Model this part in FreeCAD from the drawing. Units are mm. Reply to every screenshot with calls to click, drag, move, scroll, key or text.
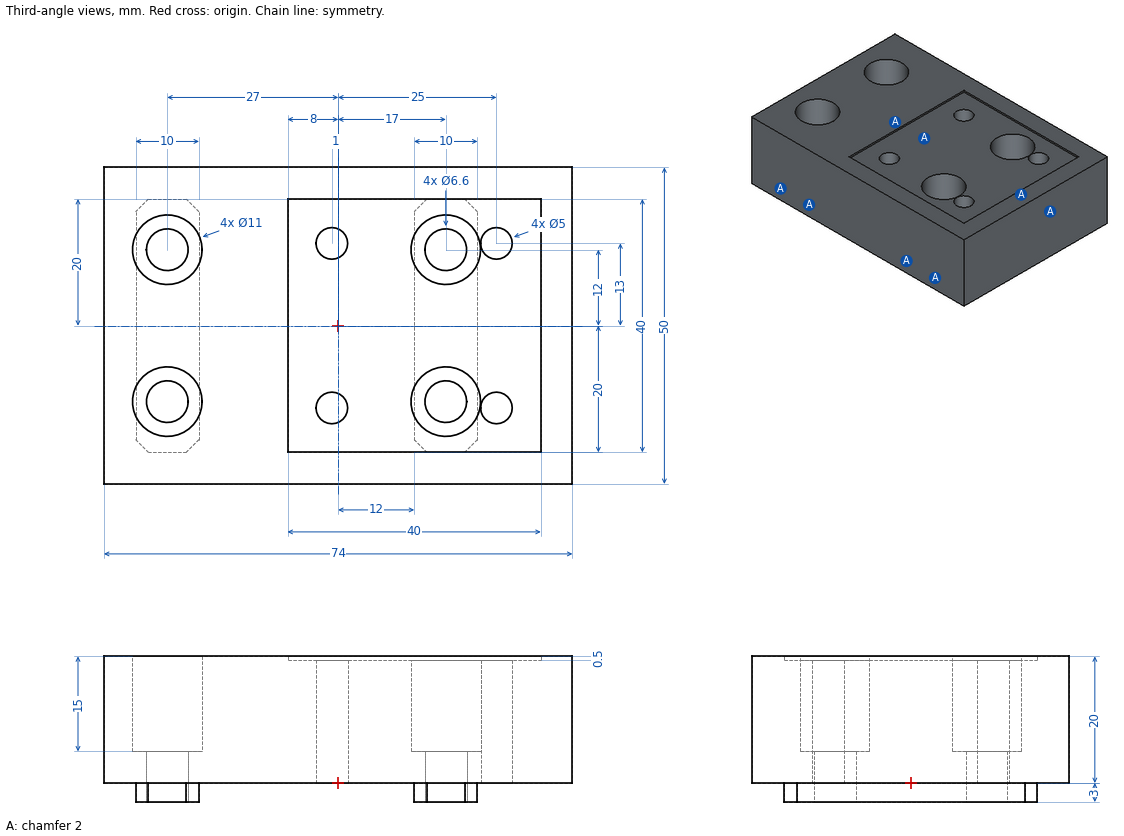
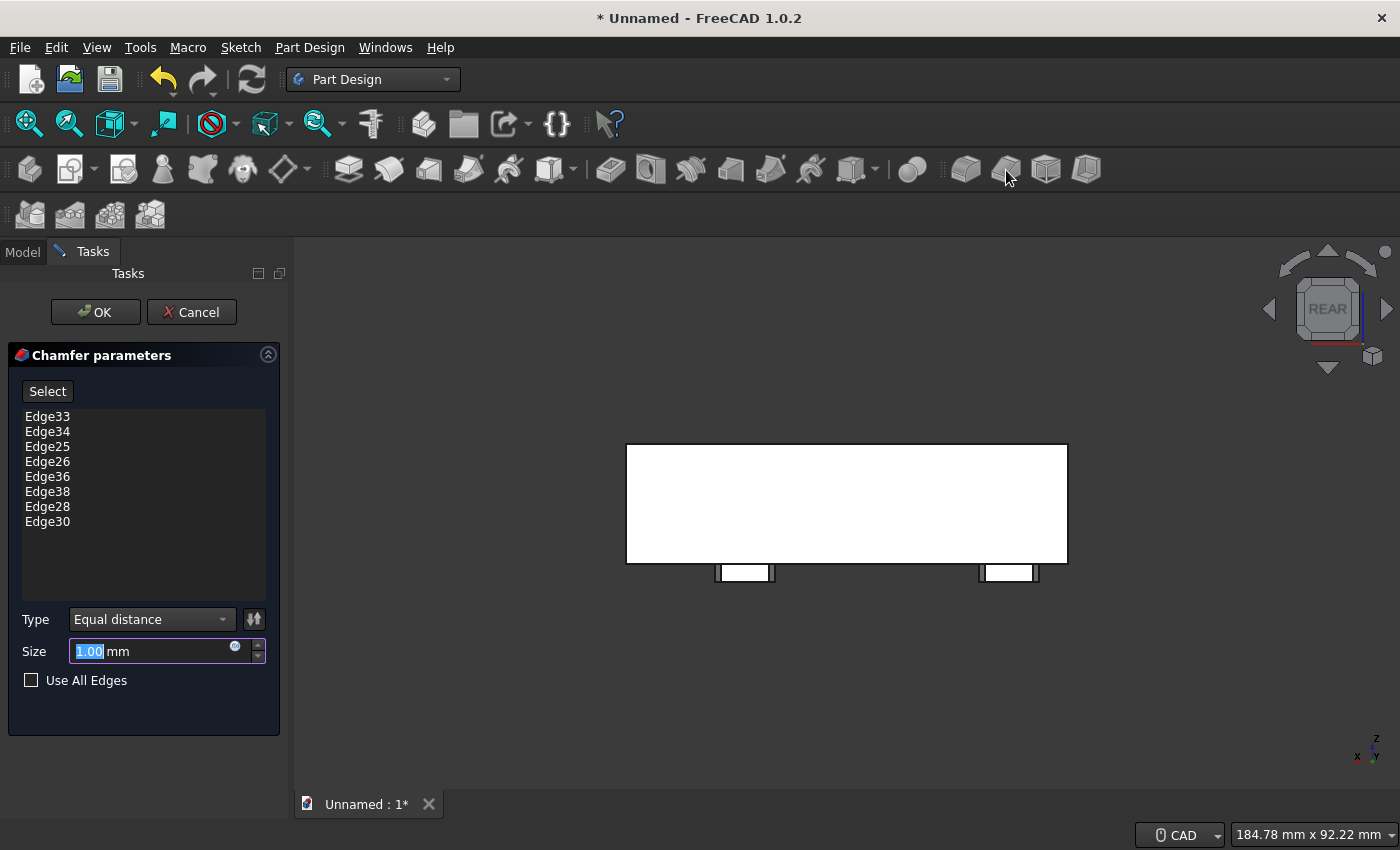
text(2)
key(Tab)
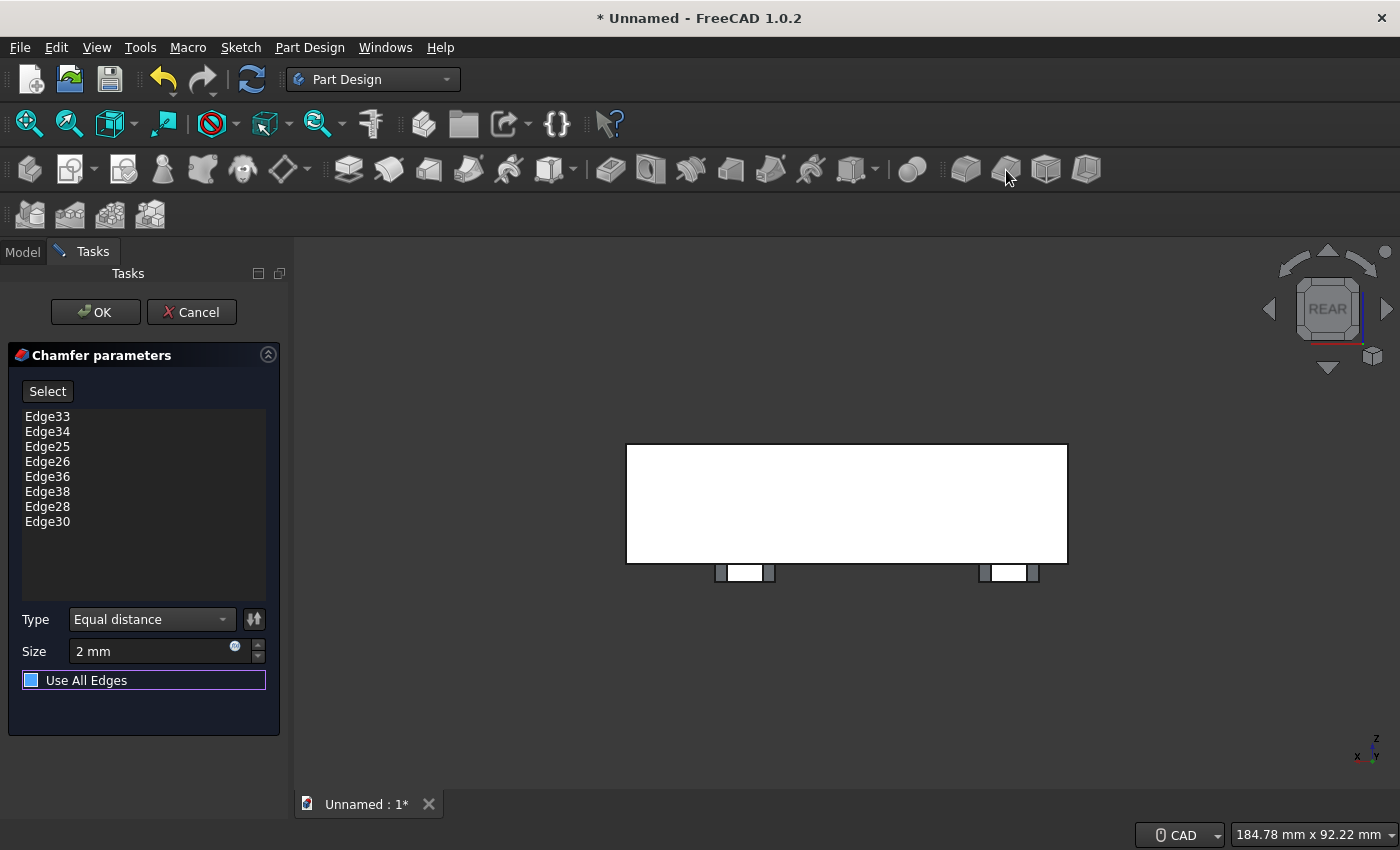
click(96, 312)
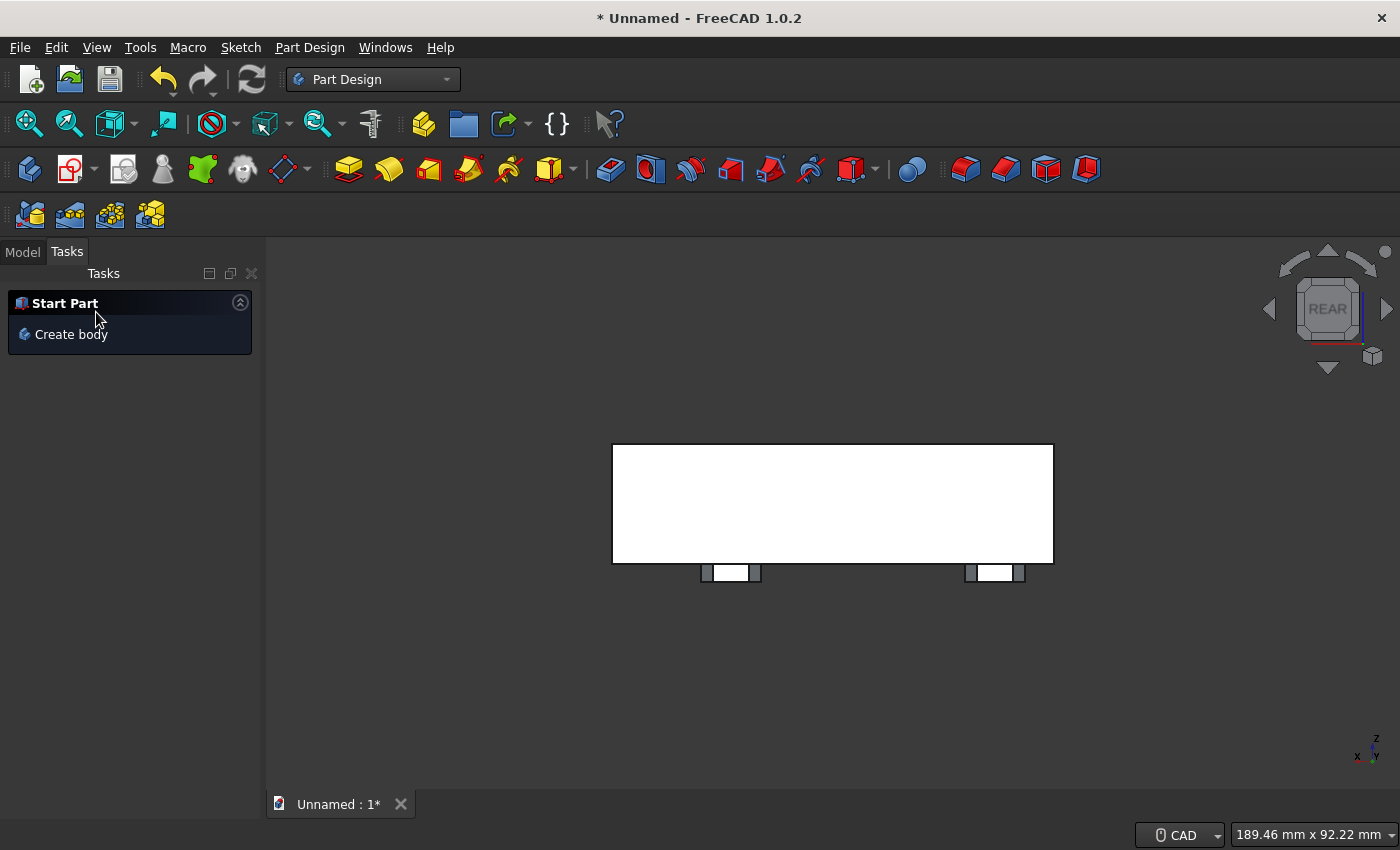
click(30, 124)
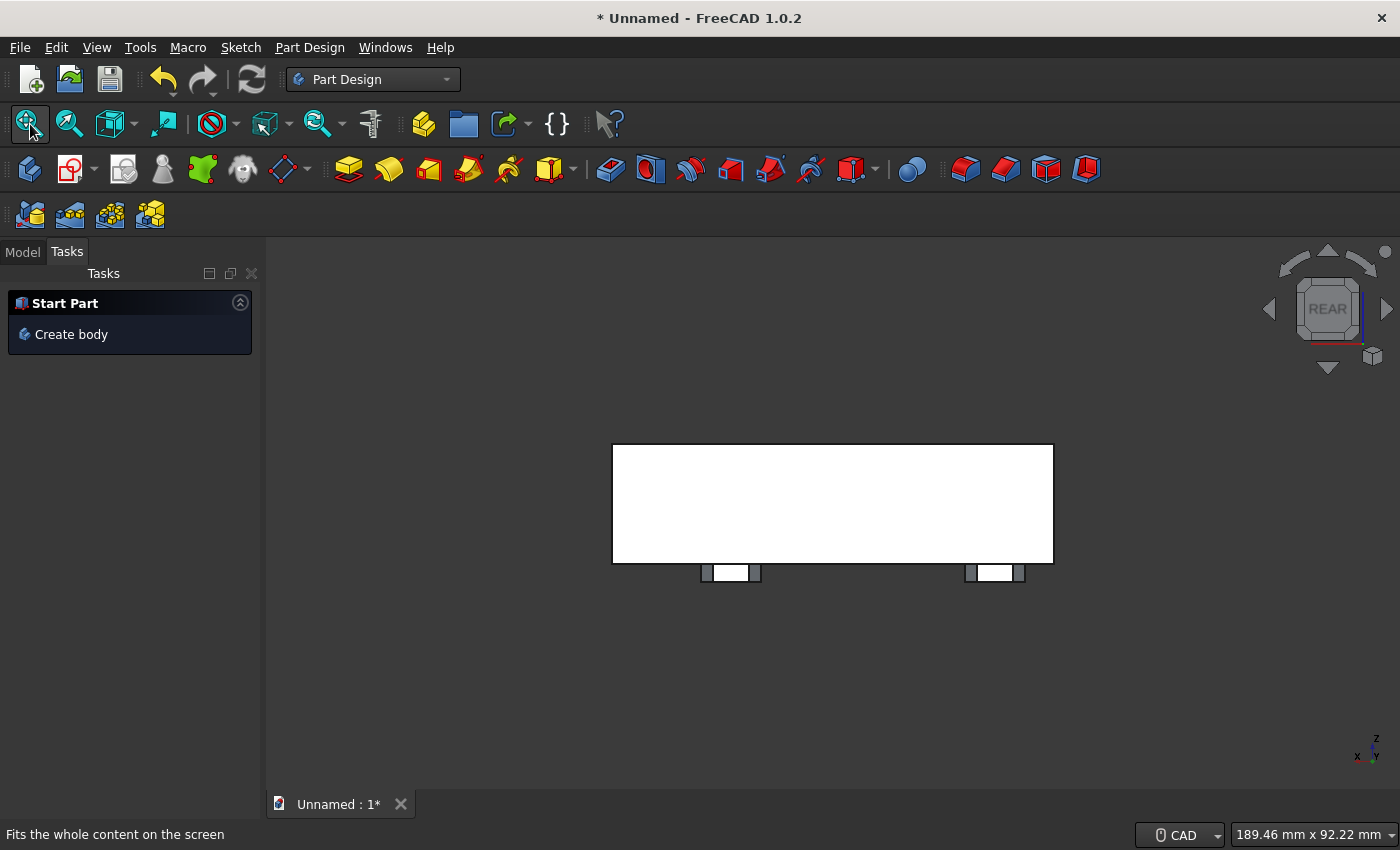
key(5)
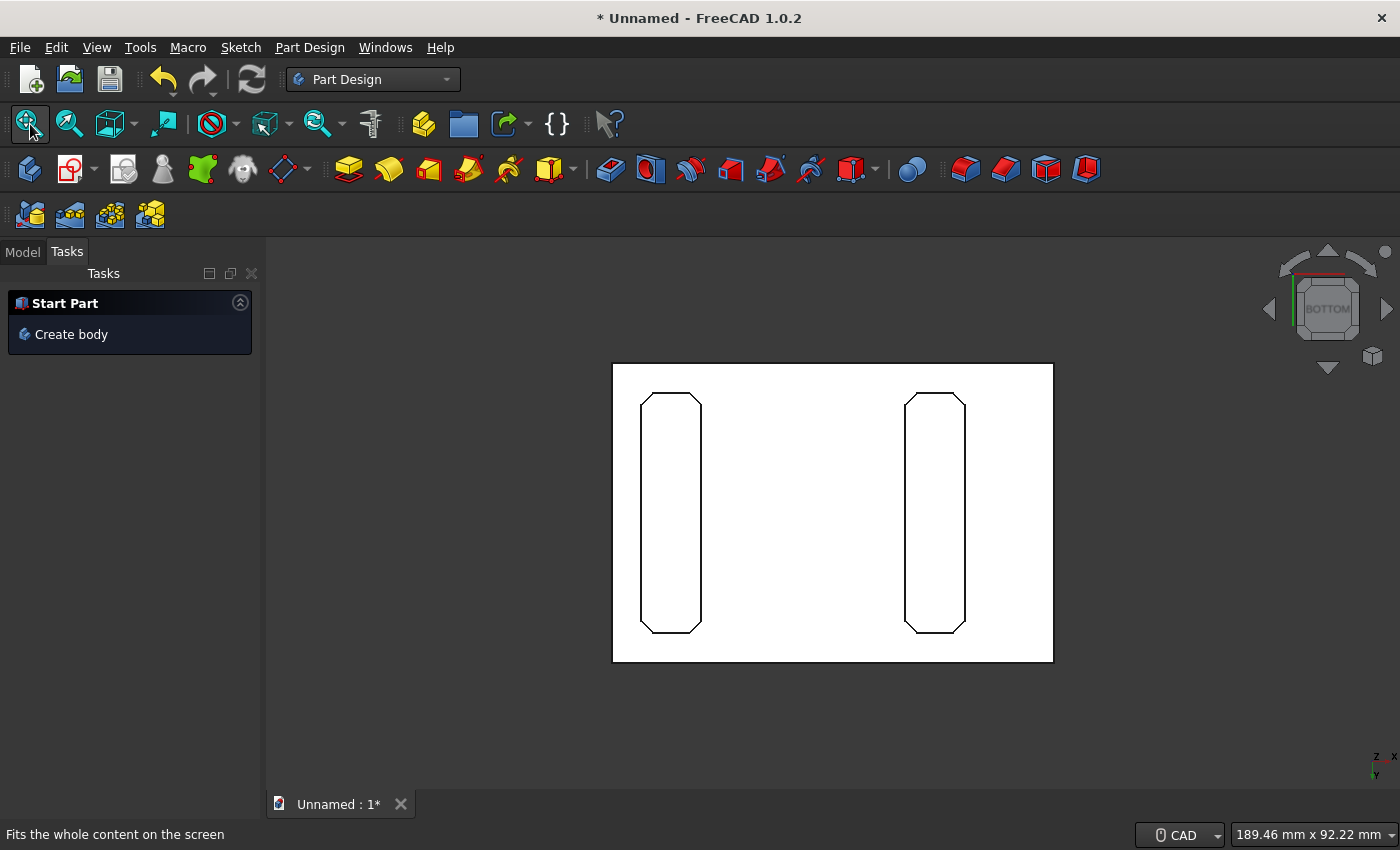
click(935, 580)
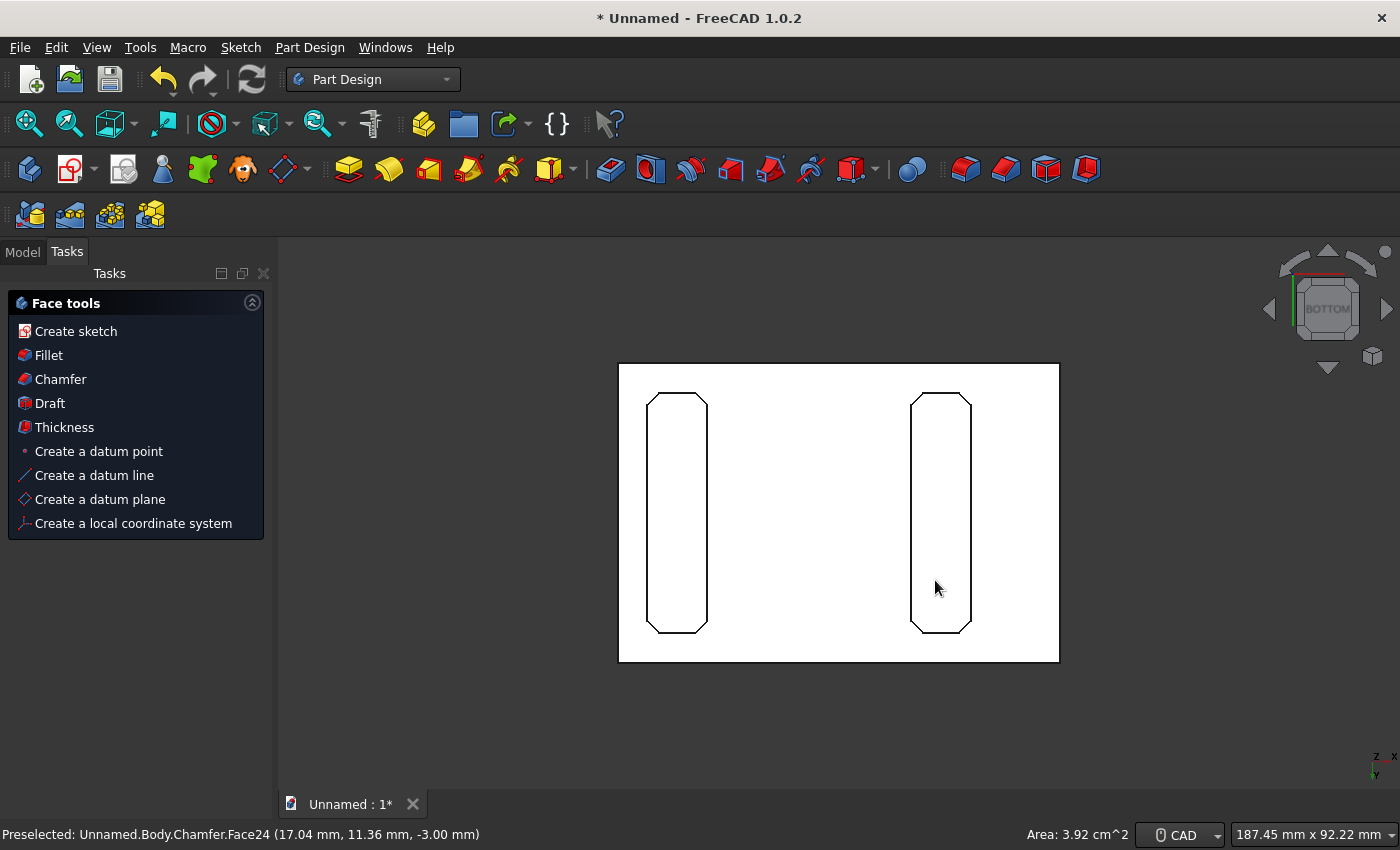
click(70, 170)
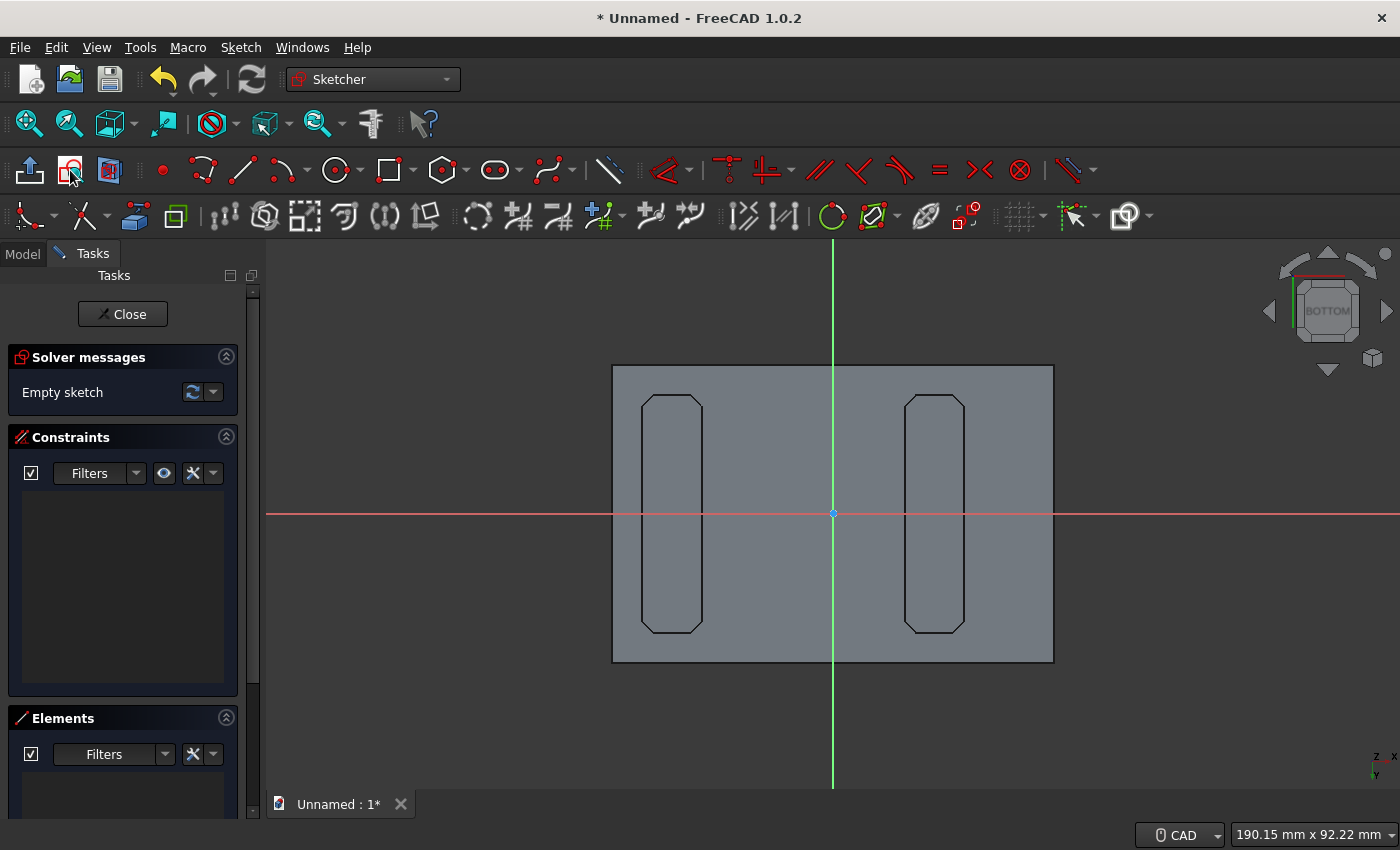
scroll(898, 514, up, 3)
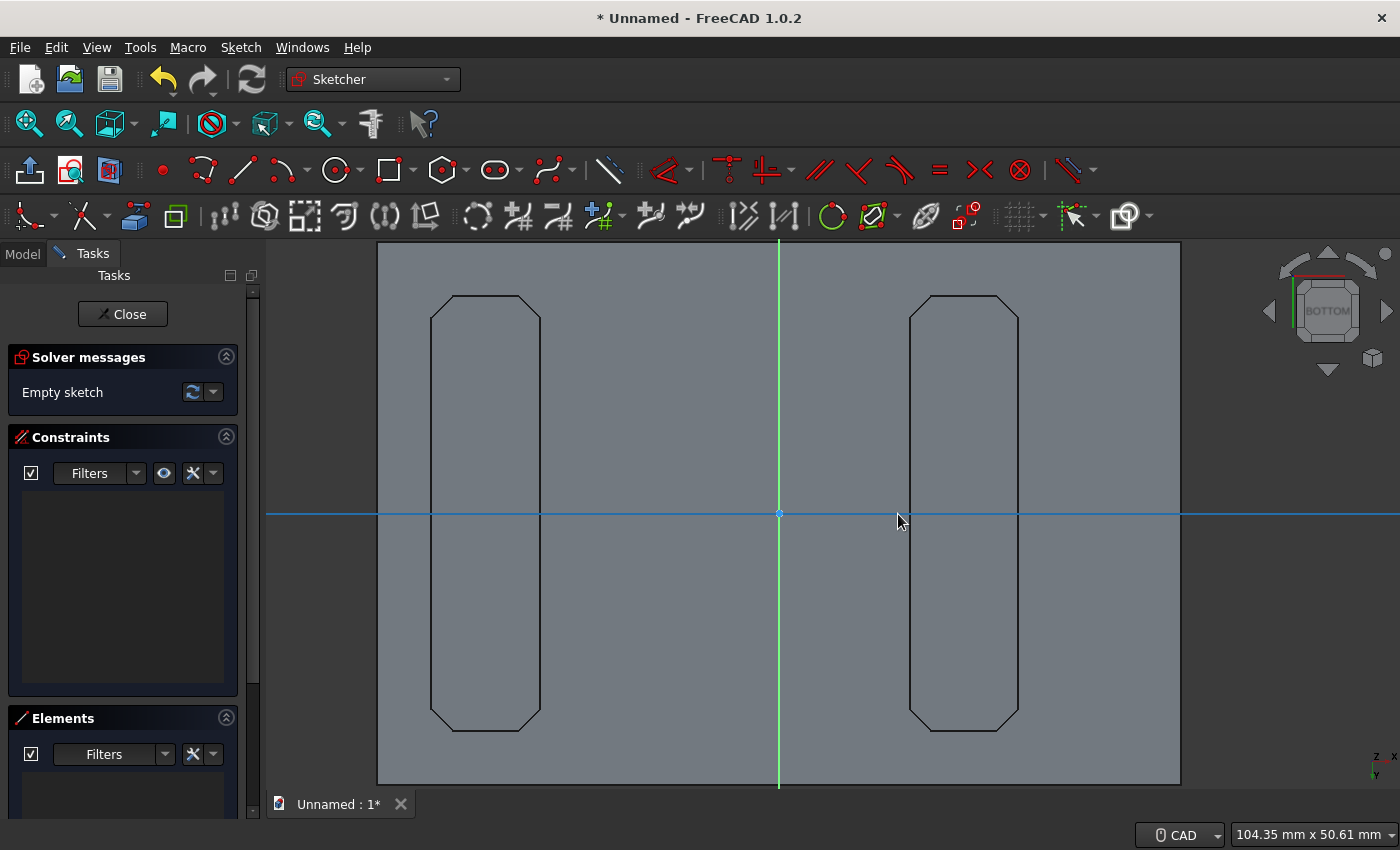
click(336, 170)